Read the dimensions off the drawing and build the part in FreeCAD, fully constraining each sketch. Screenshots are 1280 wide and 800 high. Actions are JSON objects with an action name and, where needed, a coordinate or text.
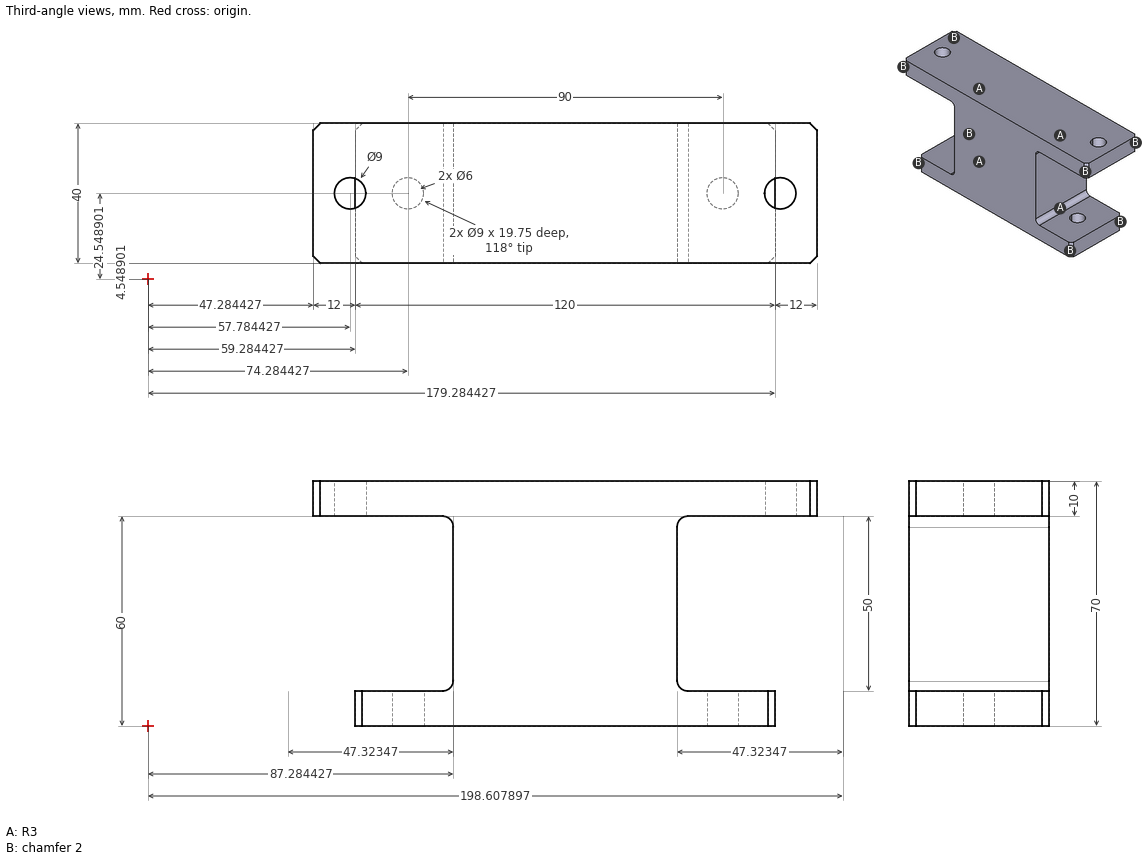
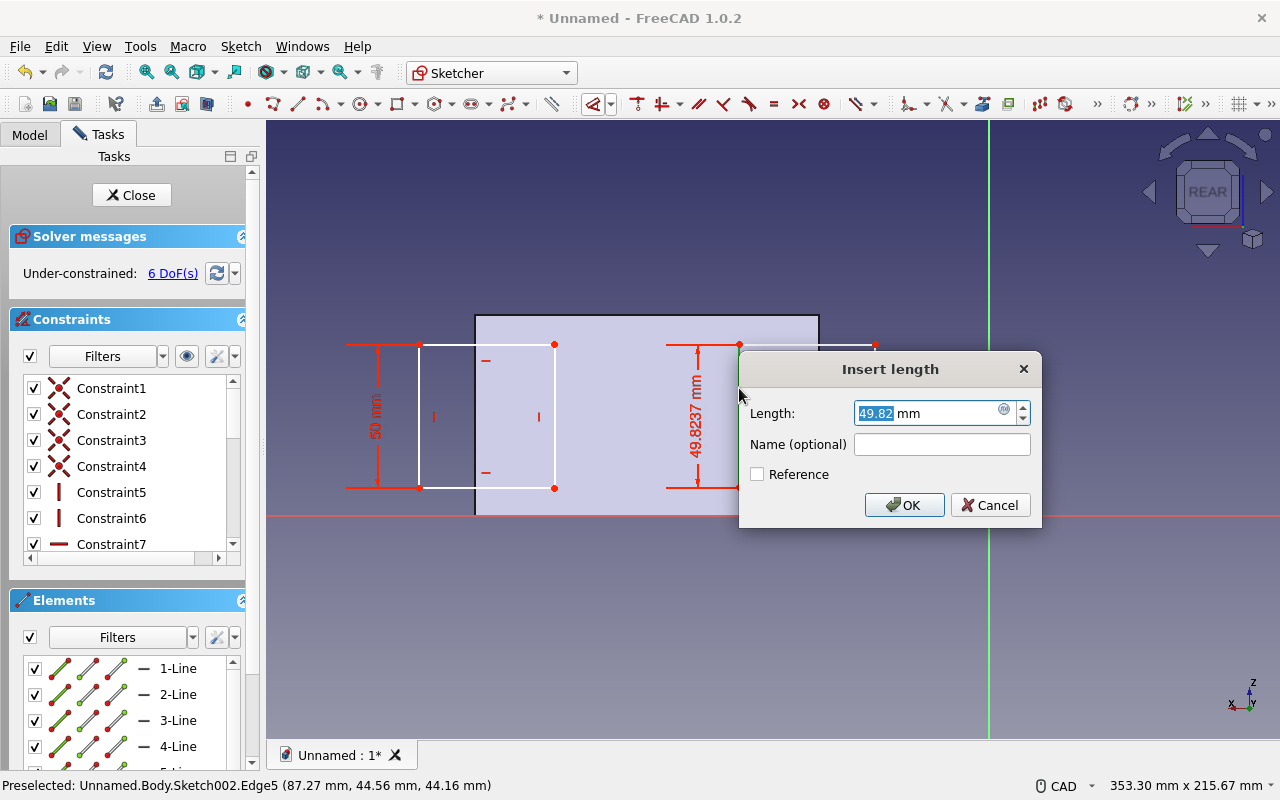
{"action": "type", "text": "50"}
{"action": "key", "text": "Return"}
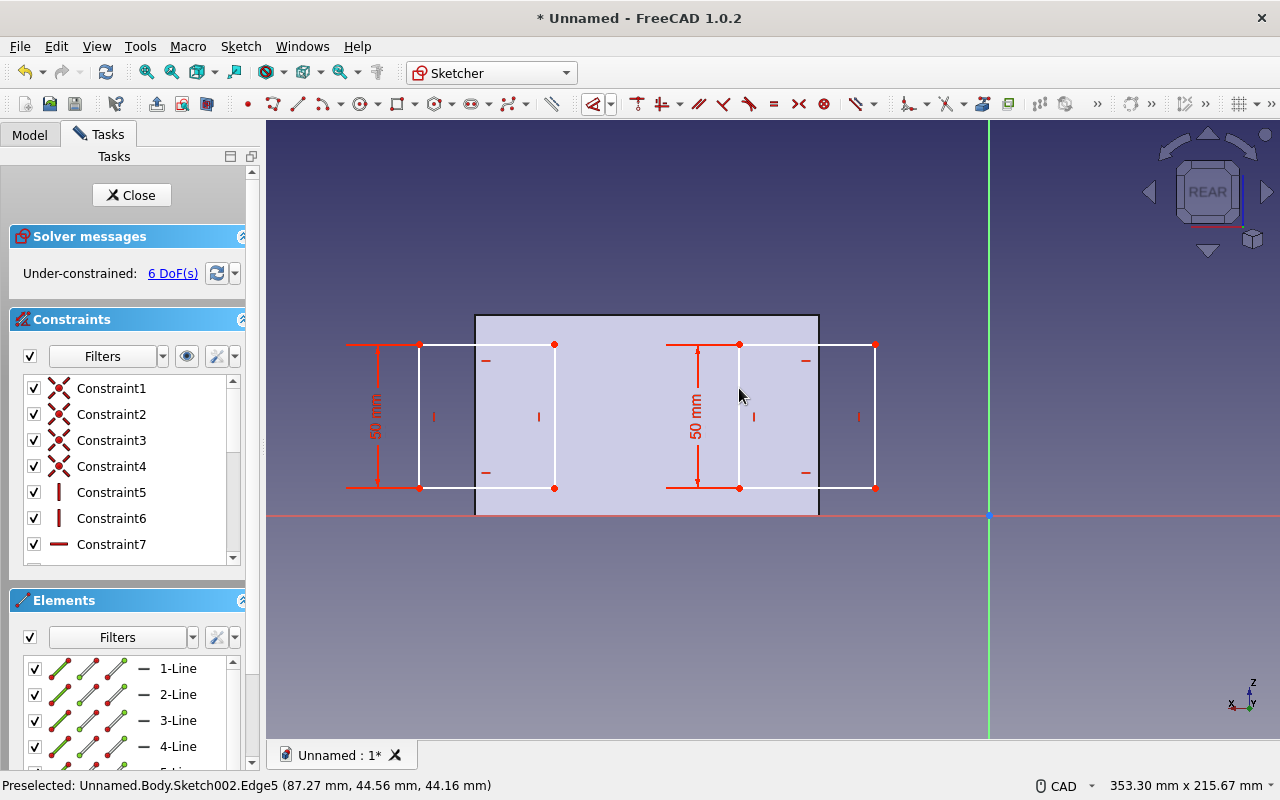
{"action": "left_click", "coordinate": [419, 345]}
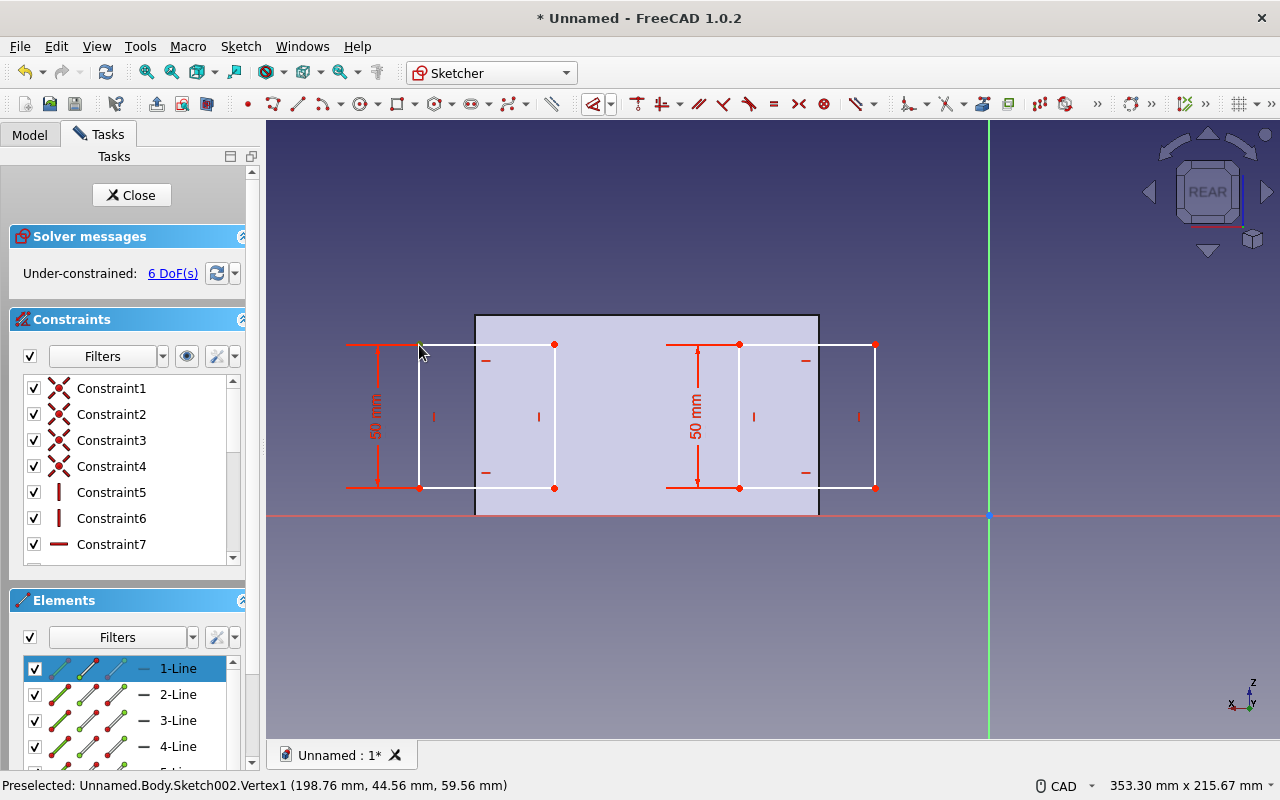
{"action": "left_click", "coordinate": [610, 104]}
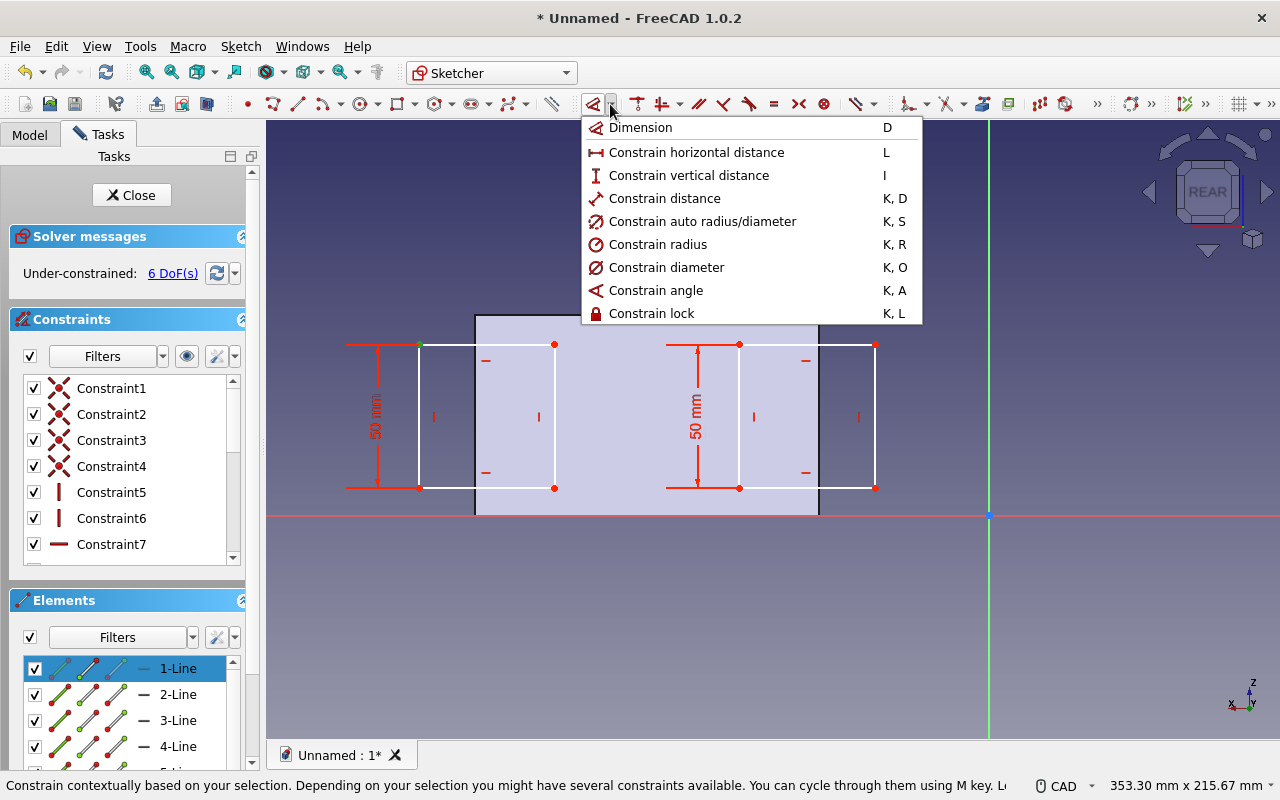
{"action": "left_click", "coordinate": [752, 176]}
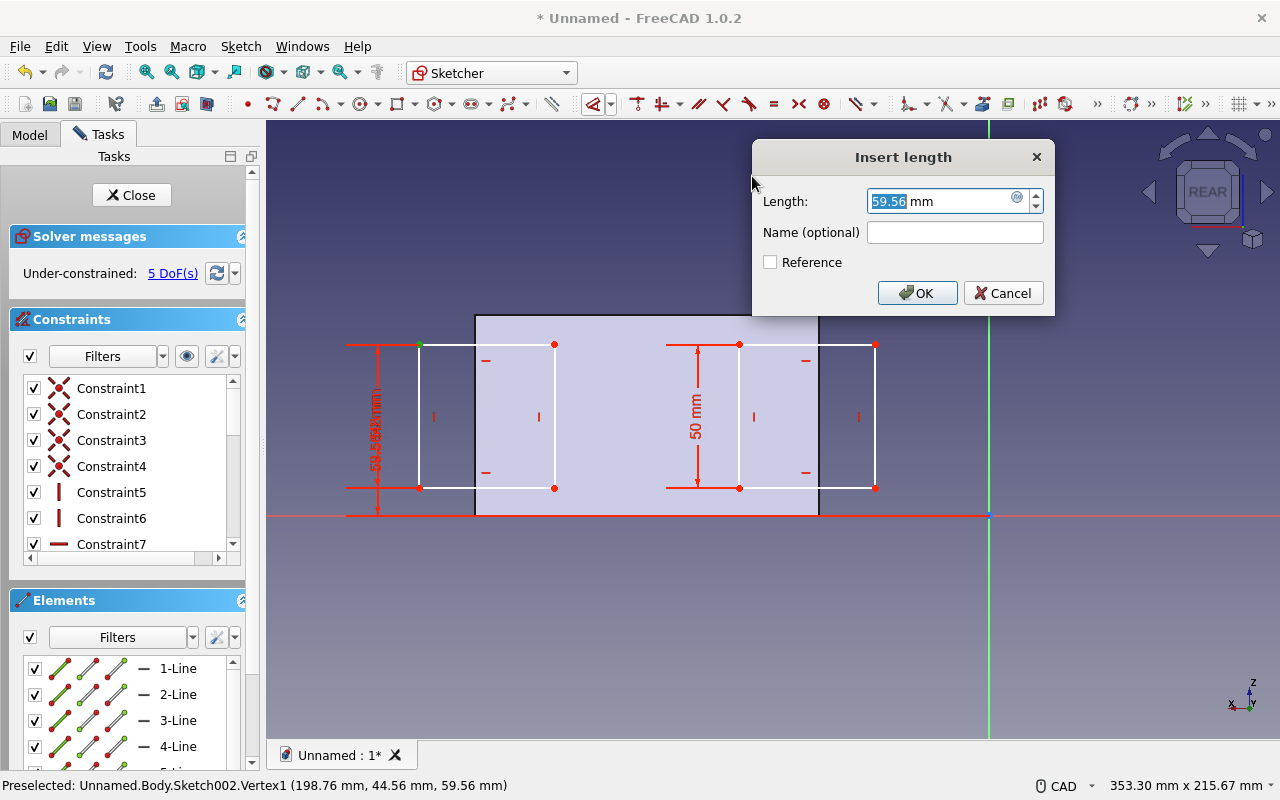
{"action": "type", "text": "60"}
{"action": "key", "text": "Return"}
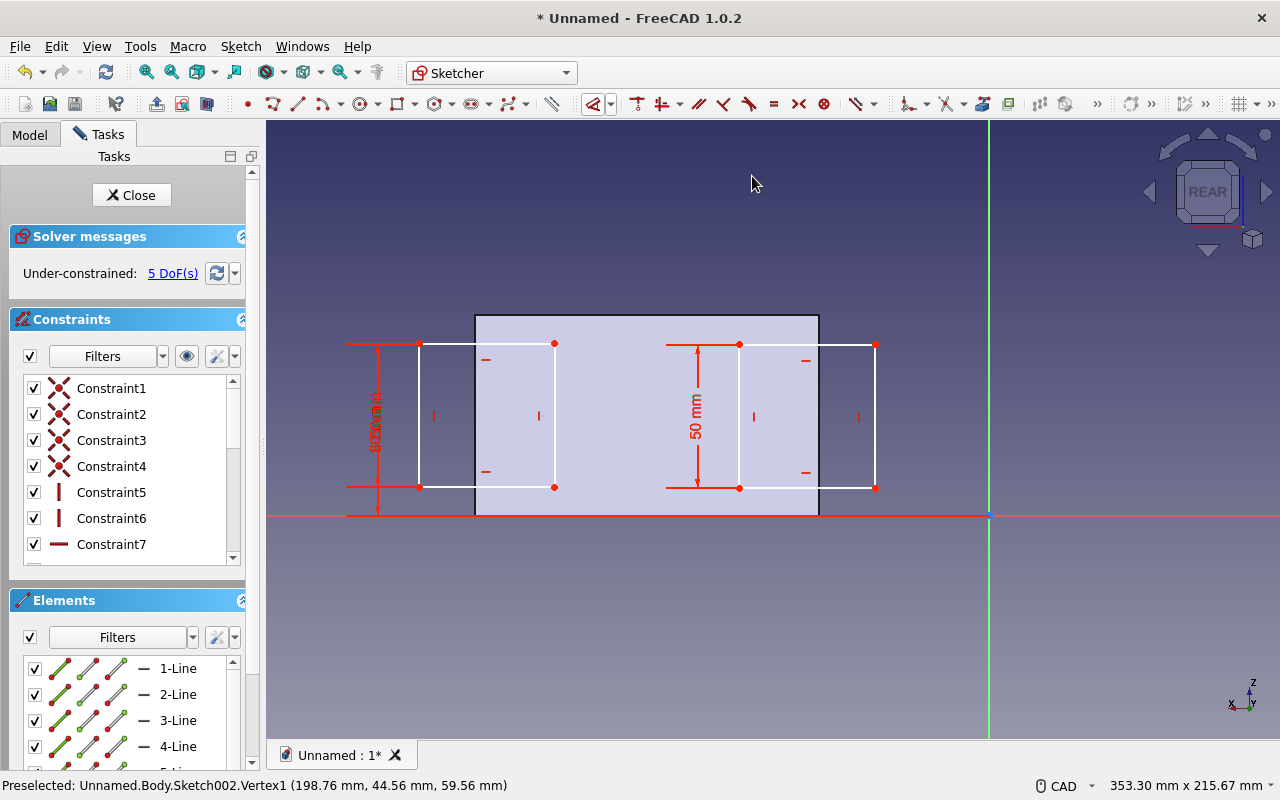
{"action": "left_click", "coordinate": [739, 345]}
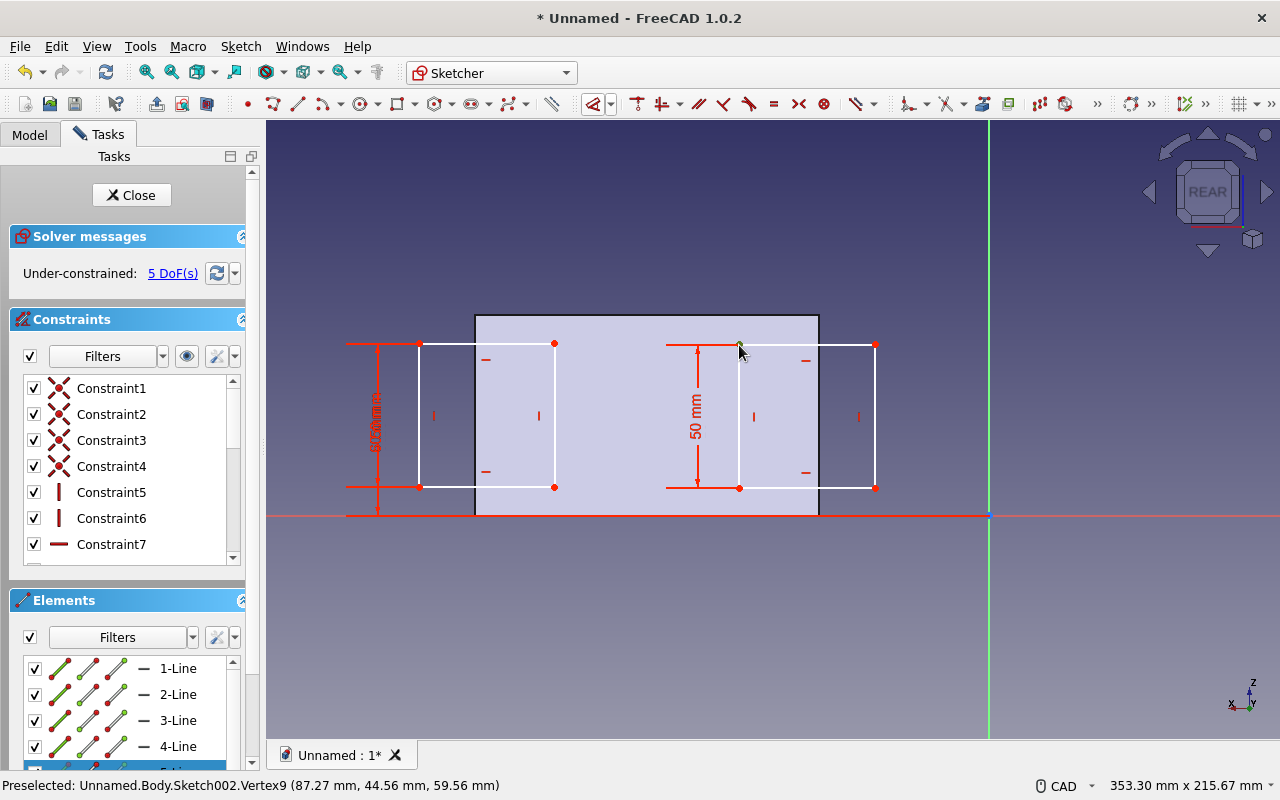
{"action": "key", "text": "i"}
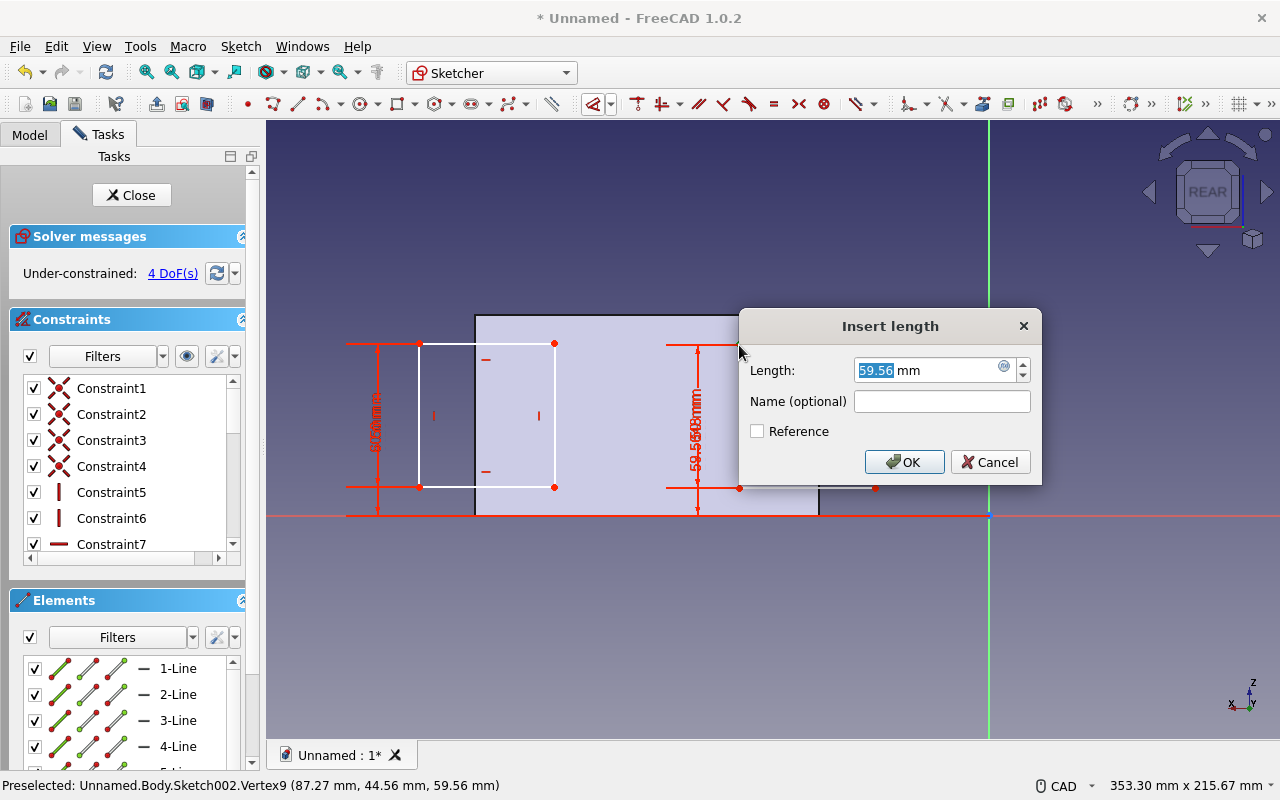
{"action": "type", "text": "60"}
{"action": "key", "text": "Return"}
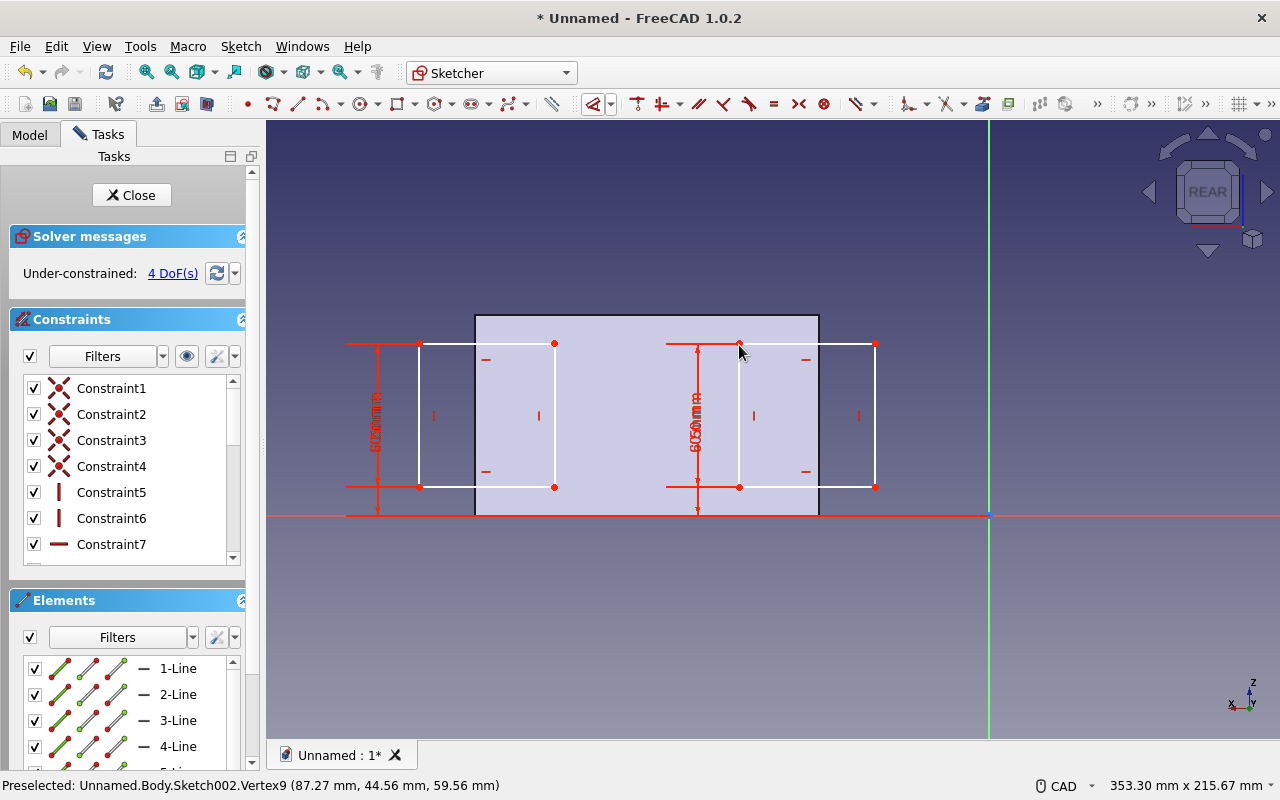
{"action": "left_click", "coordinate": [460, 487]}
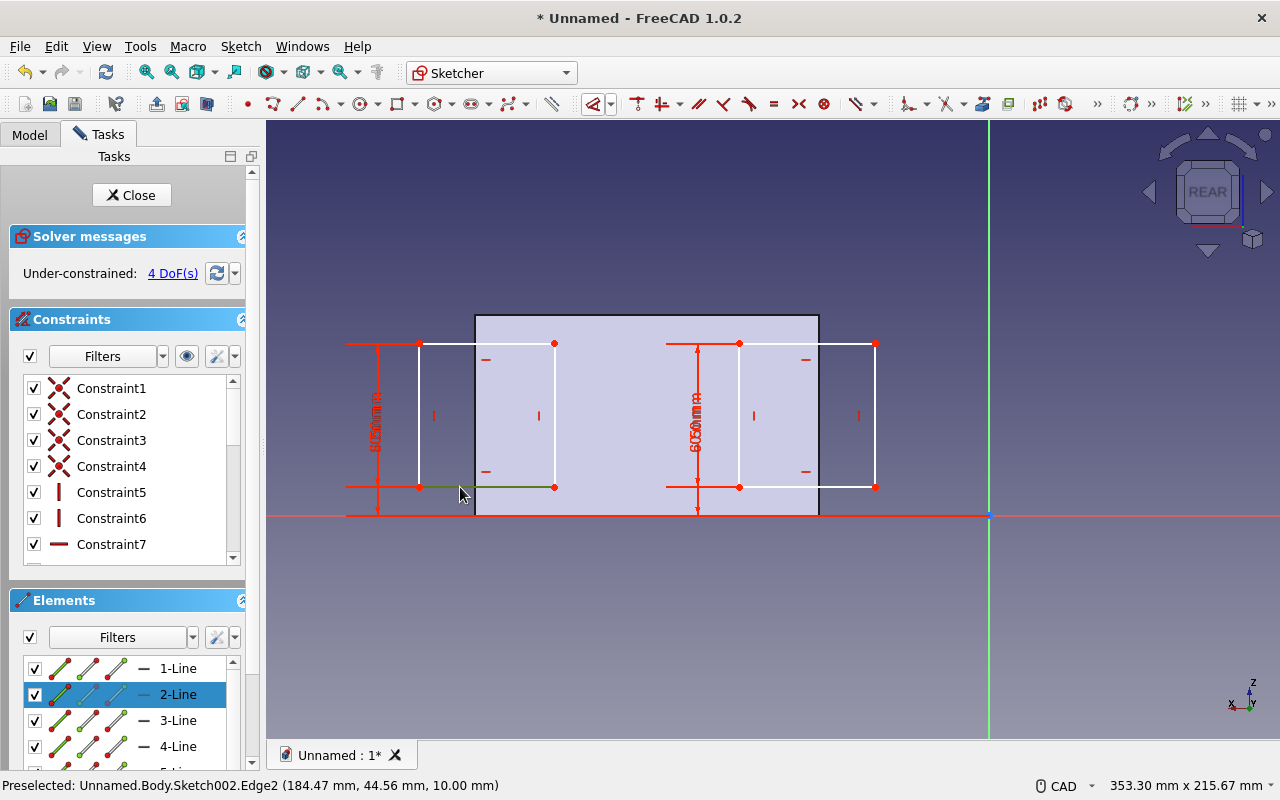
{"action": "key", "text": "l"}